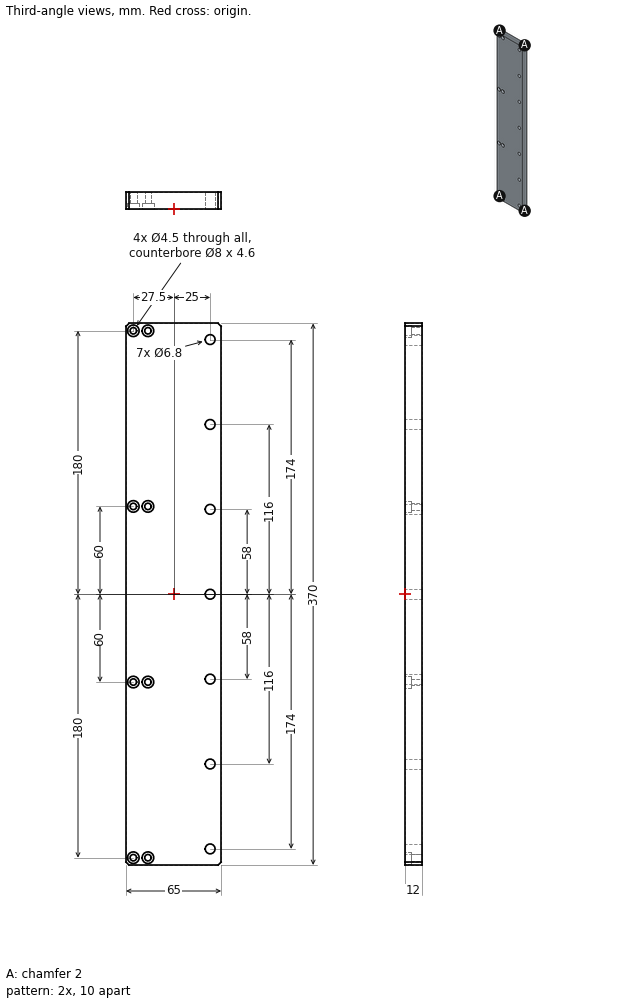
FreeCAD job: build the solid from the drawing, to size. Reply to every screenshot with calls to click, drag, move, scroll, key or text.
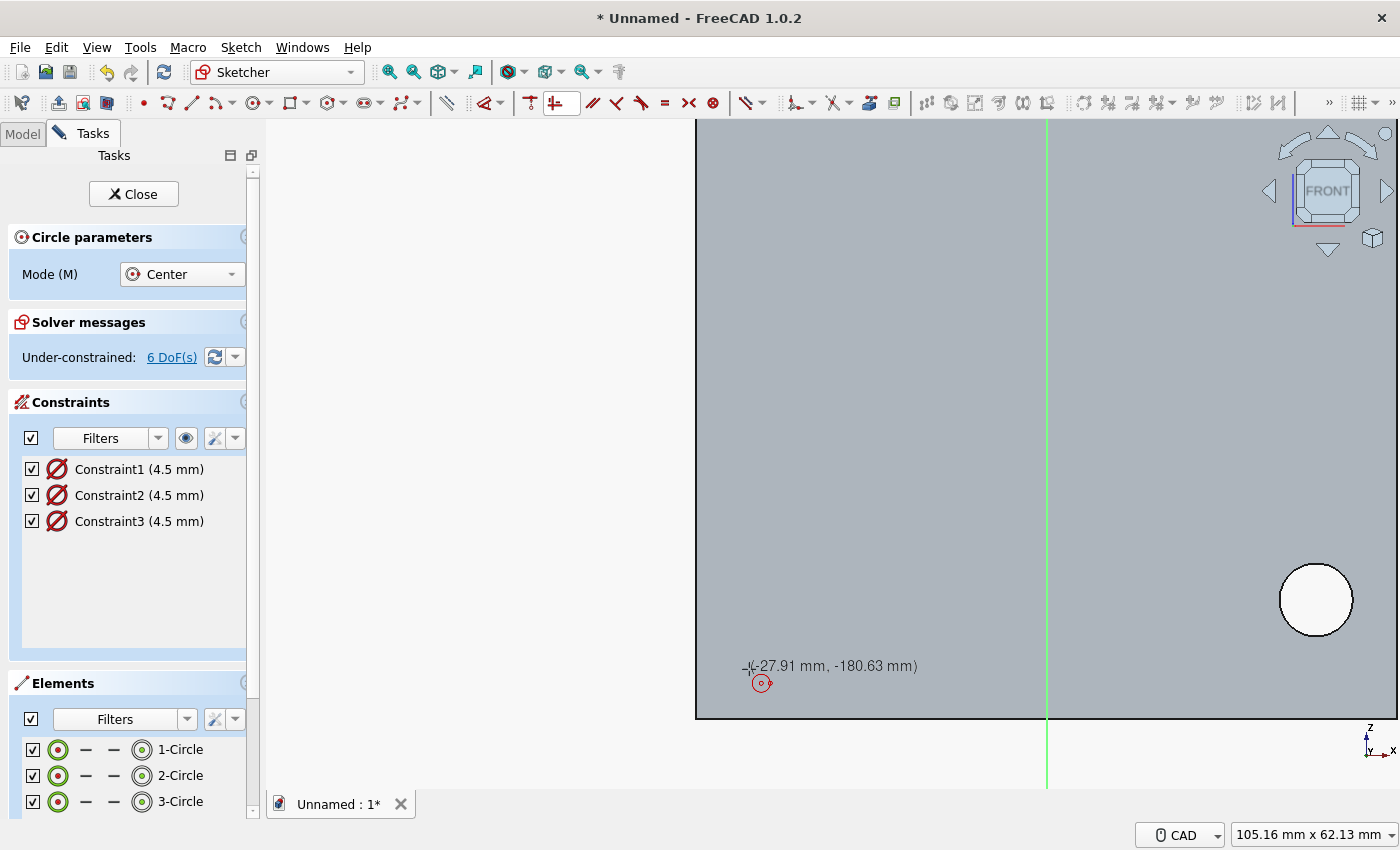
scroll(749, 670, down, 11)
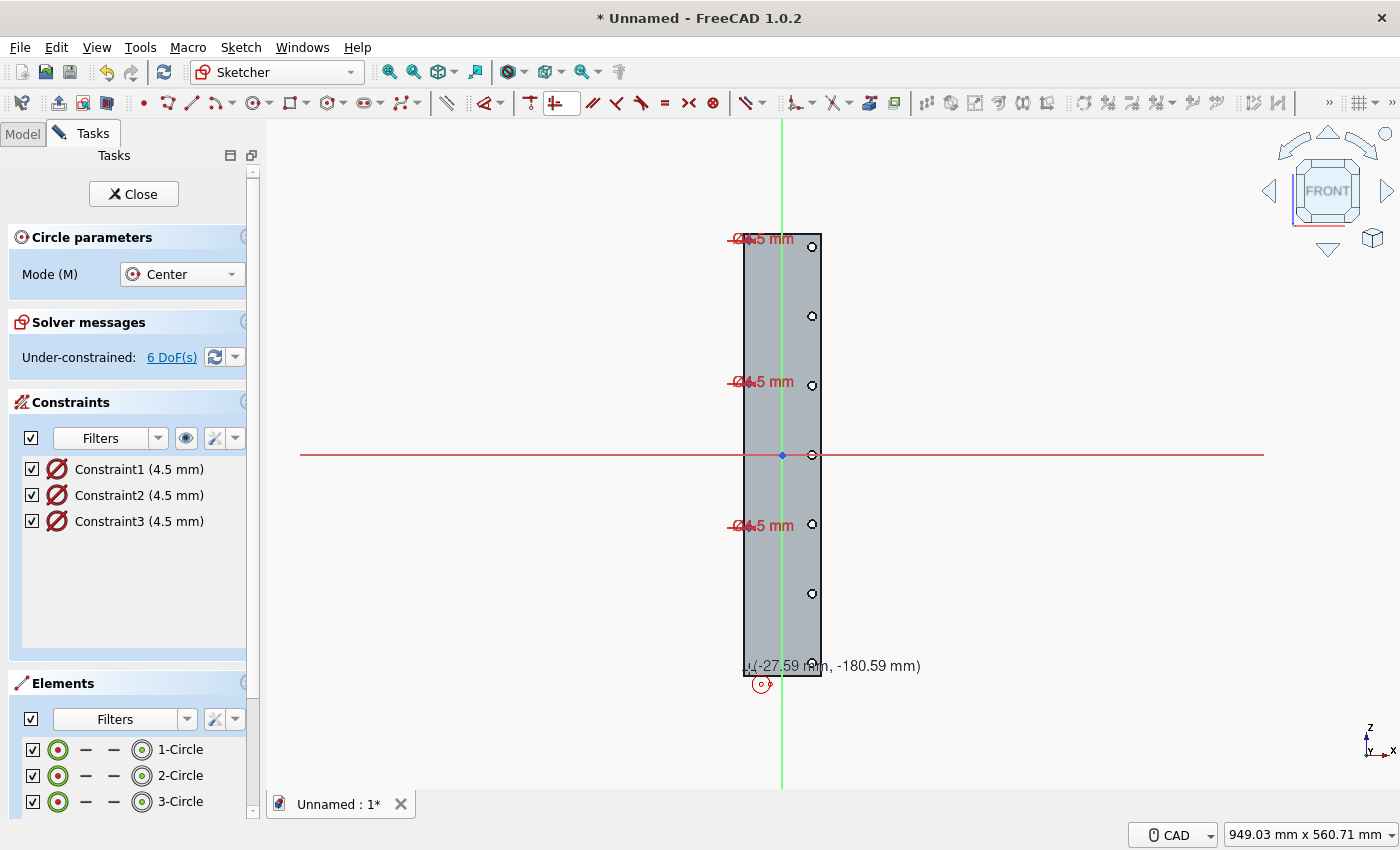
click(749, 670)
move(751, 668)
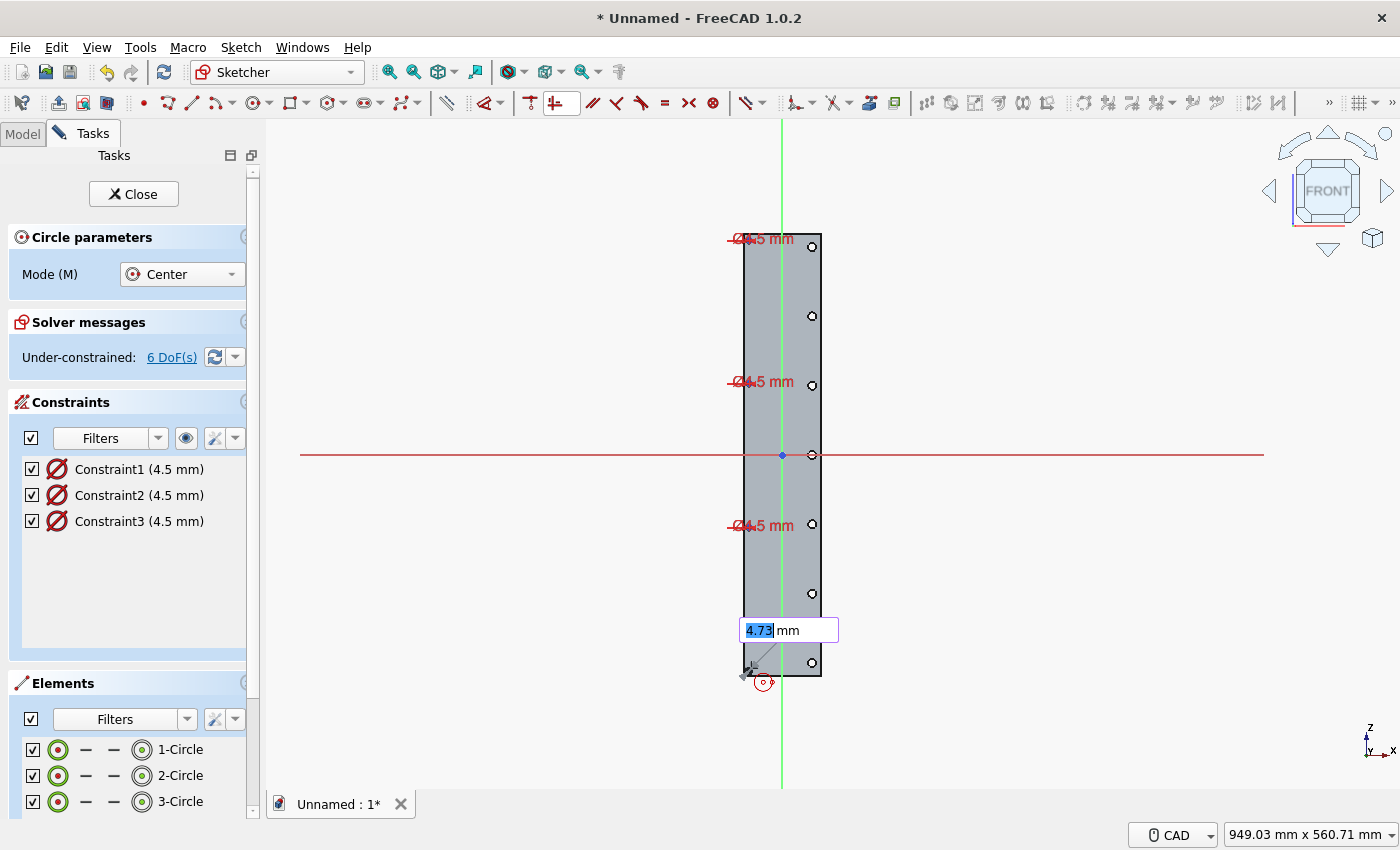
text(4.5)
key(Return)
key(Escape)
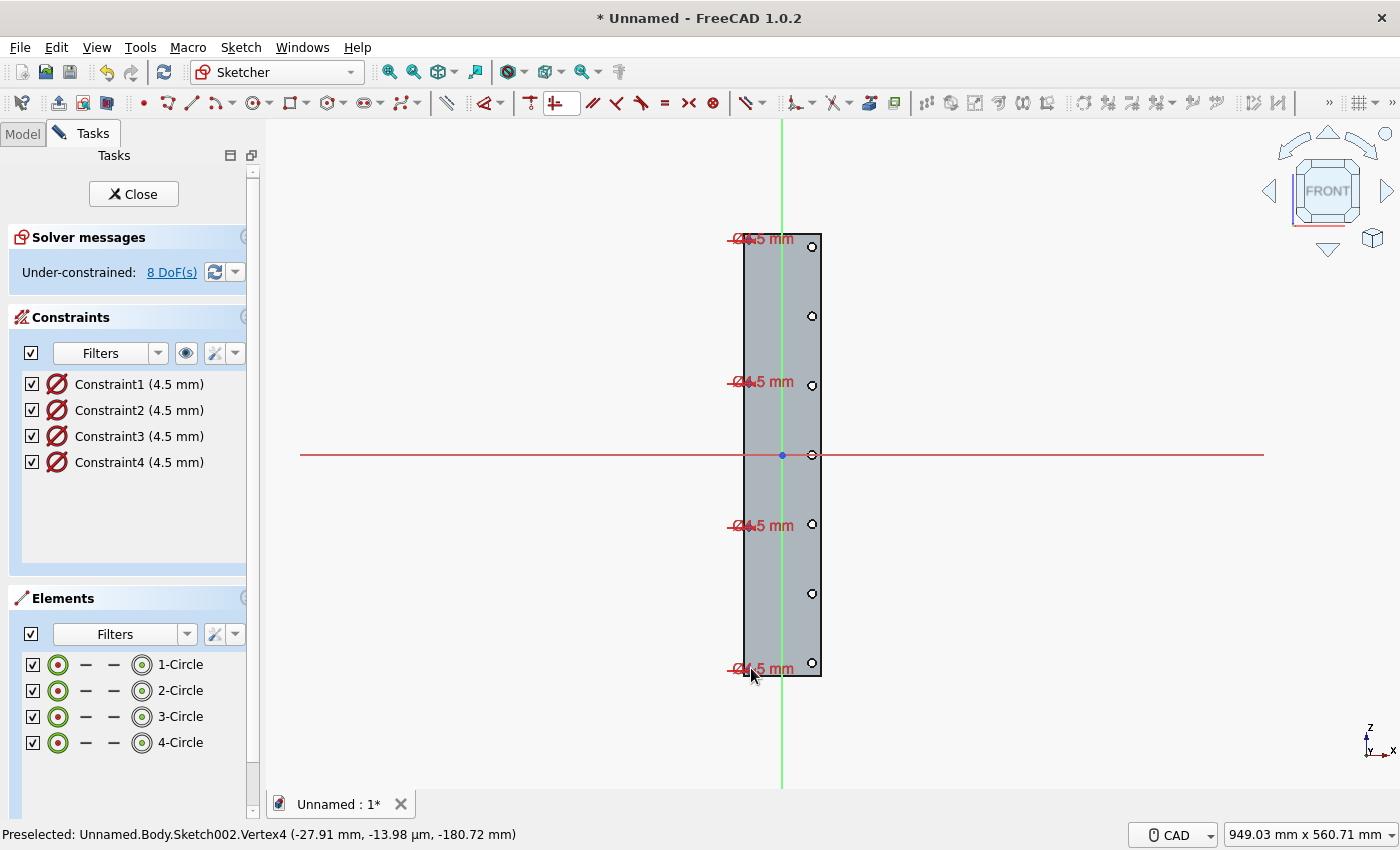
click(749, 241)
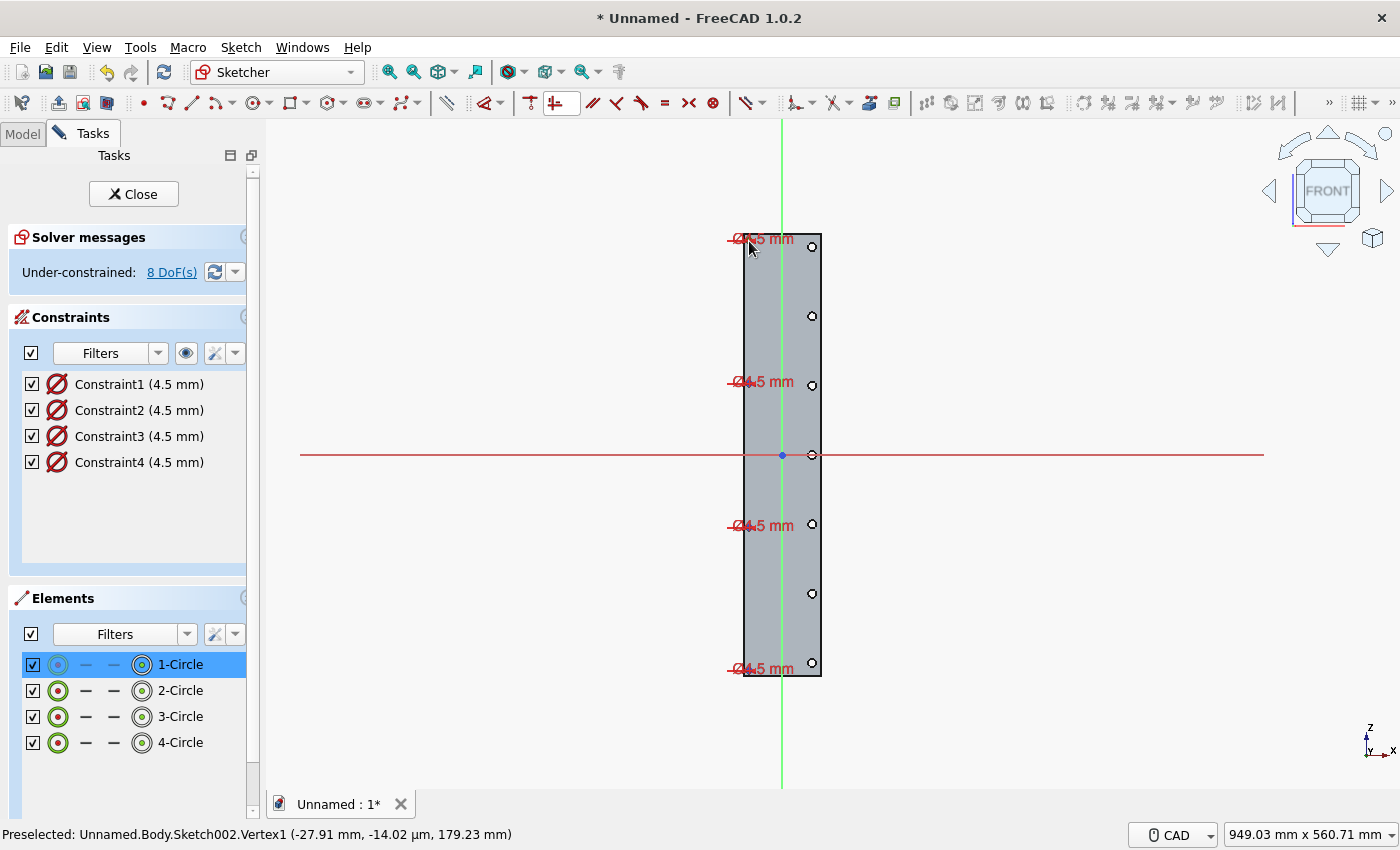
click(749, 384)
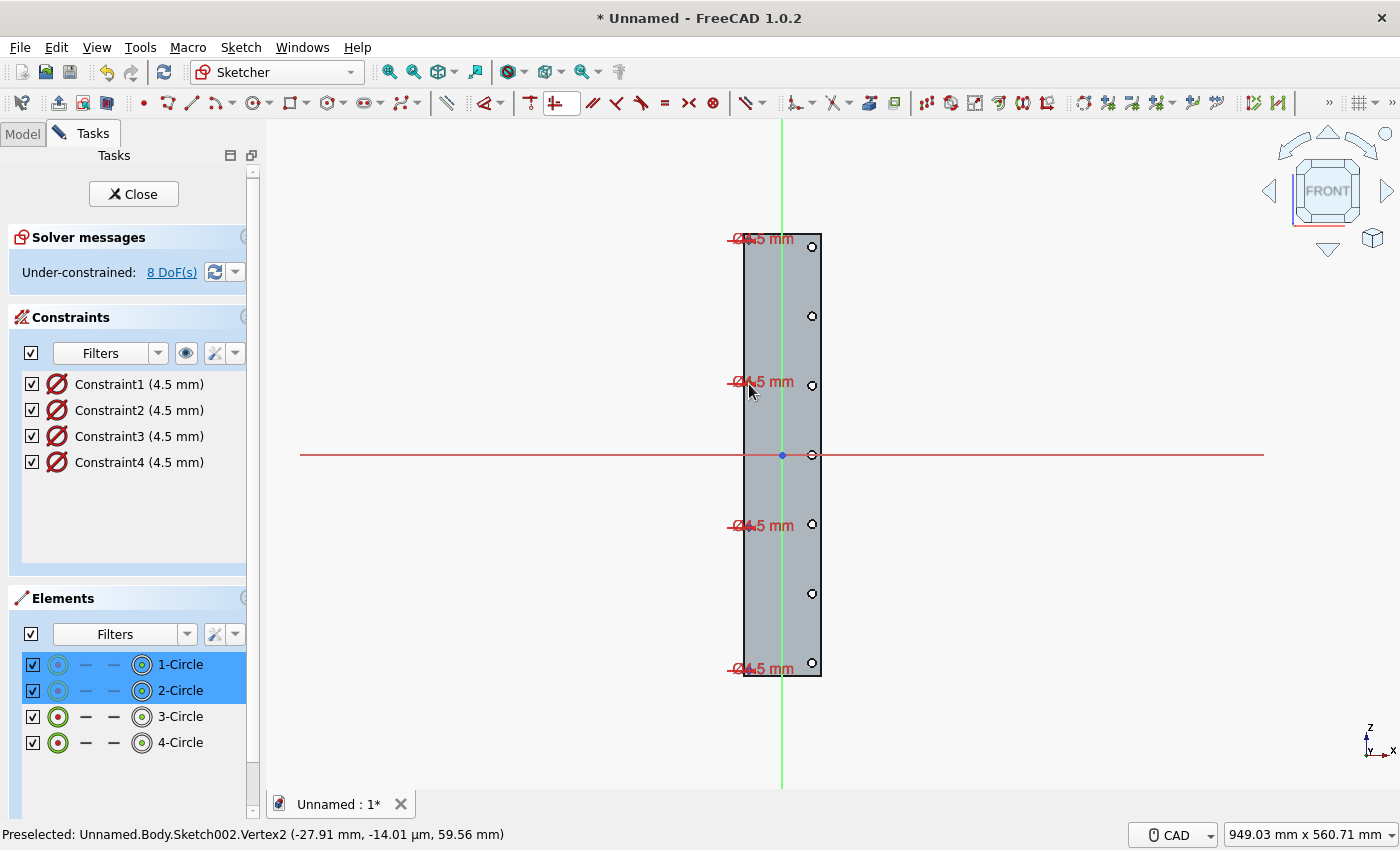
key(v)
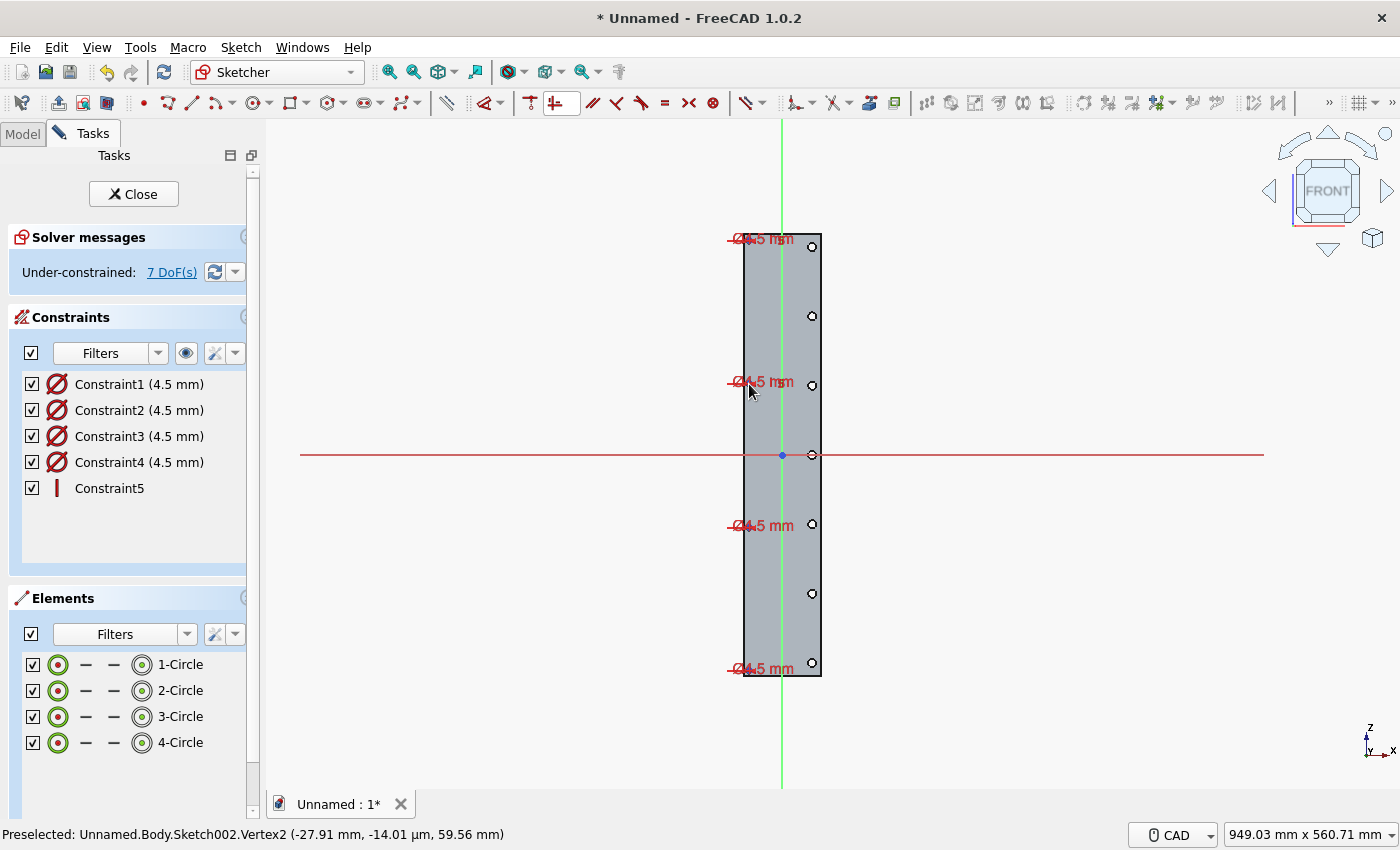
click(749, 384)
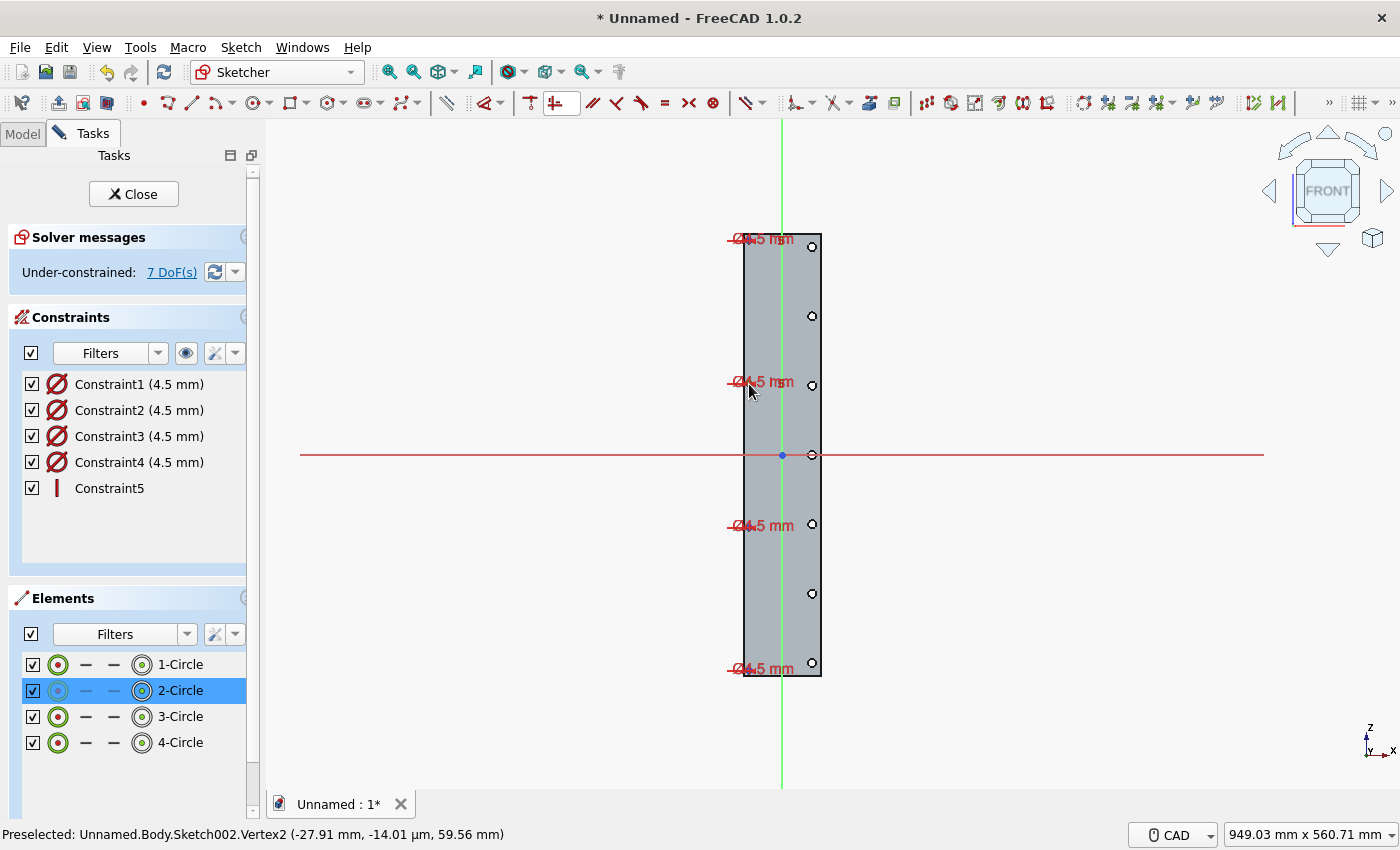
click(749, 528)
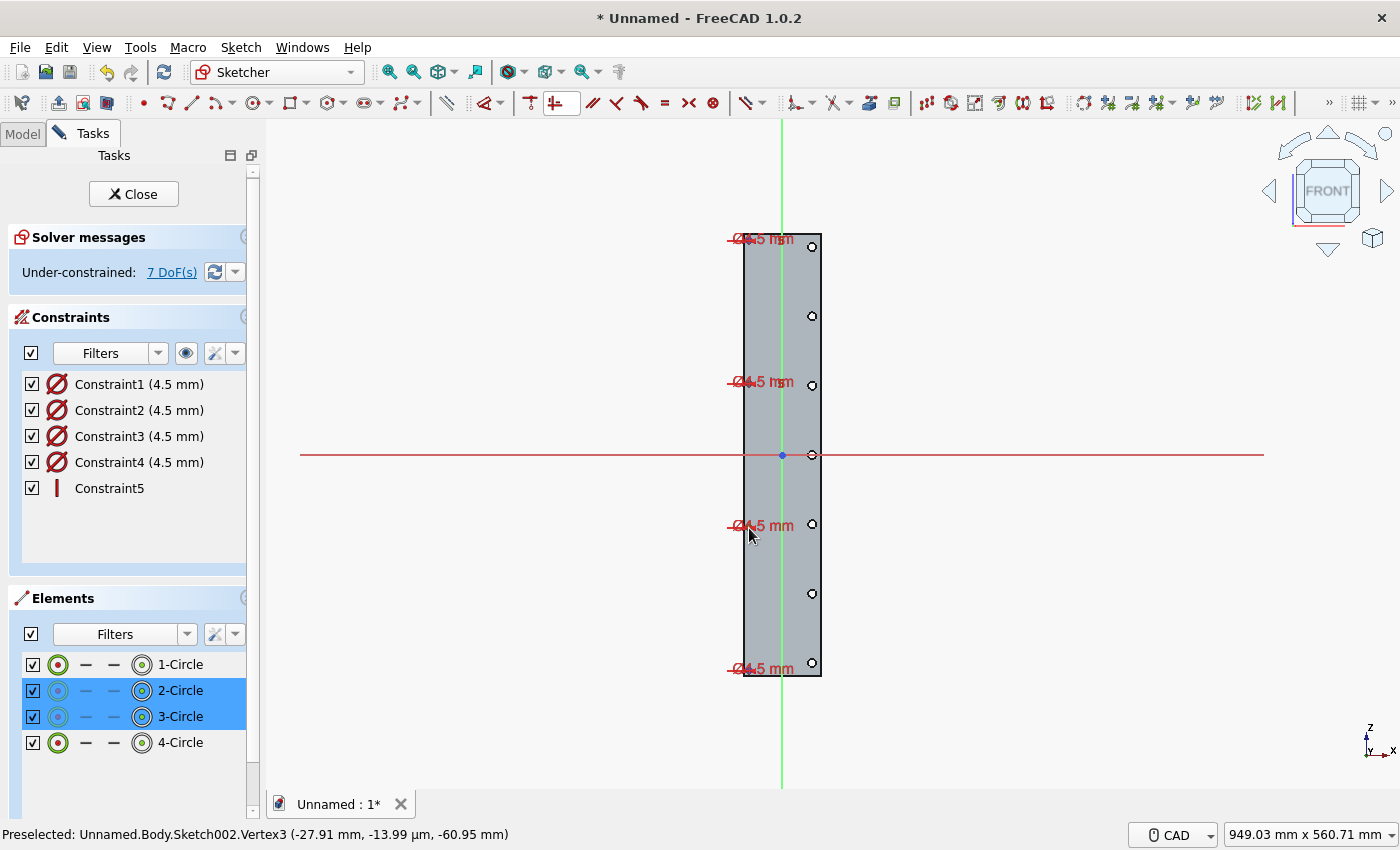
key(v)